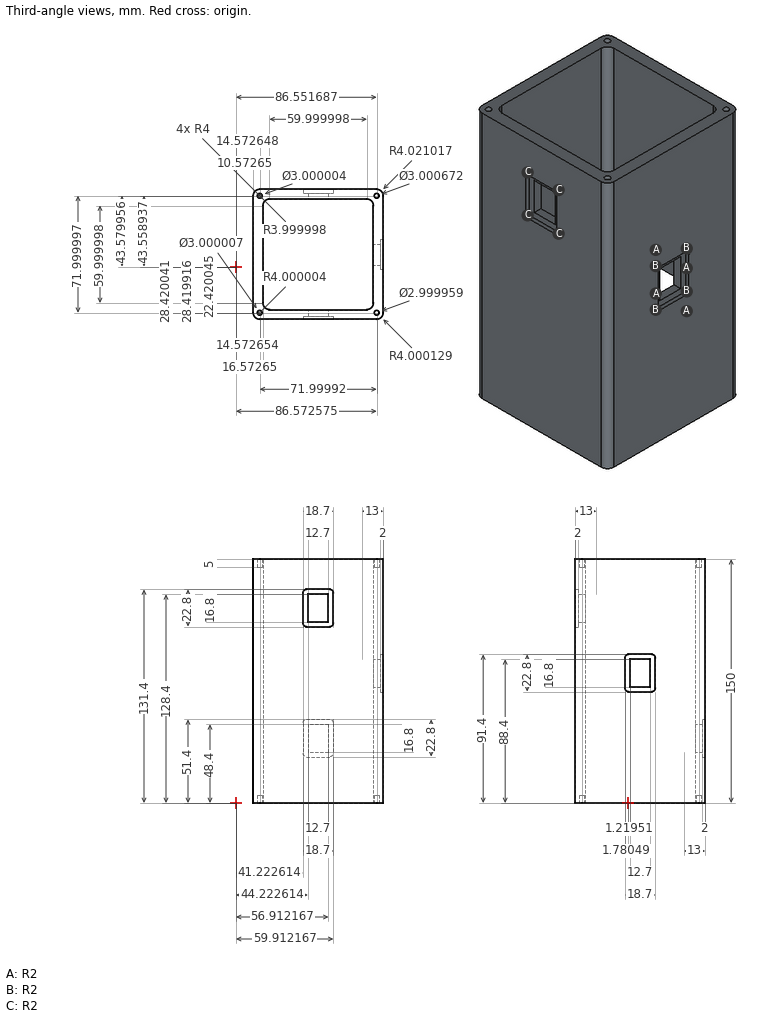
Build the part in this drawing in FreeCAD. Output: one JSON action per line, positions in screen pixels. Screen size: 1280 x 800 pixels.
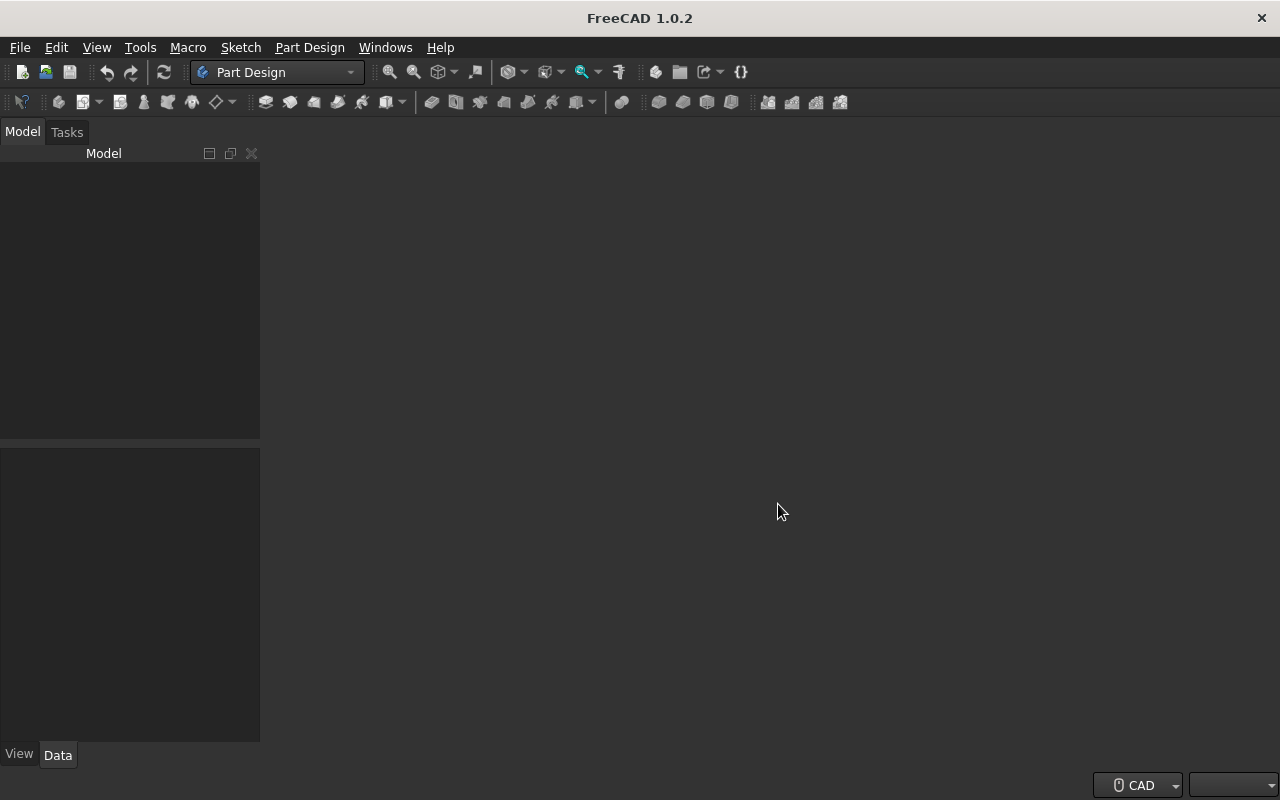
{"action": "left_click", "coordinate": [22, 72]}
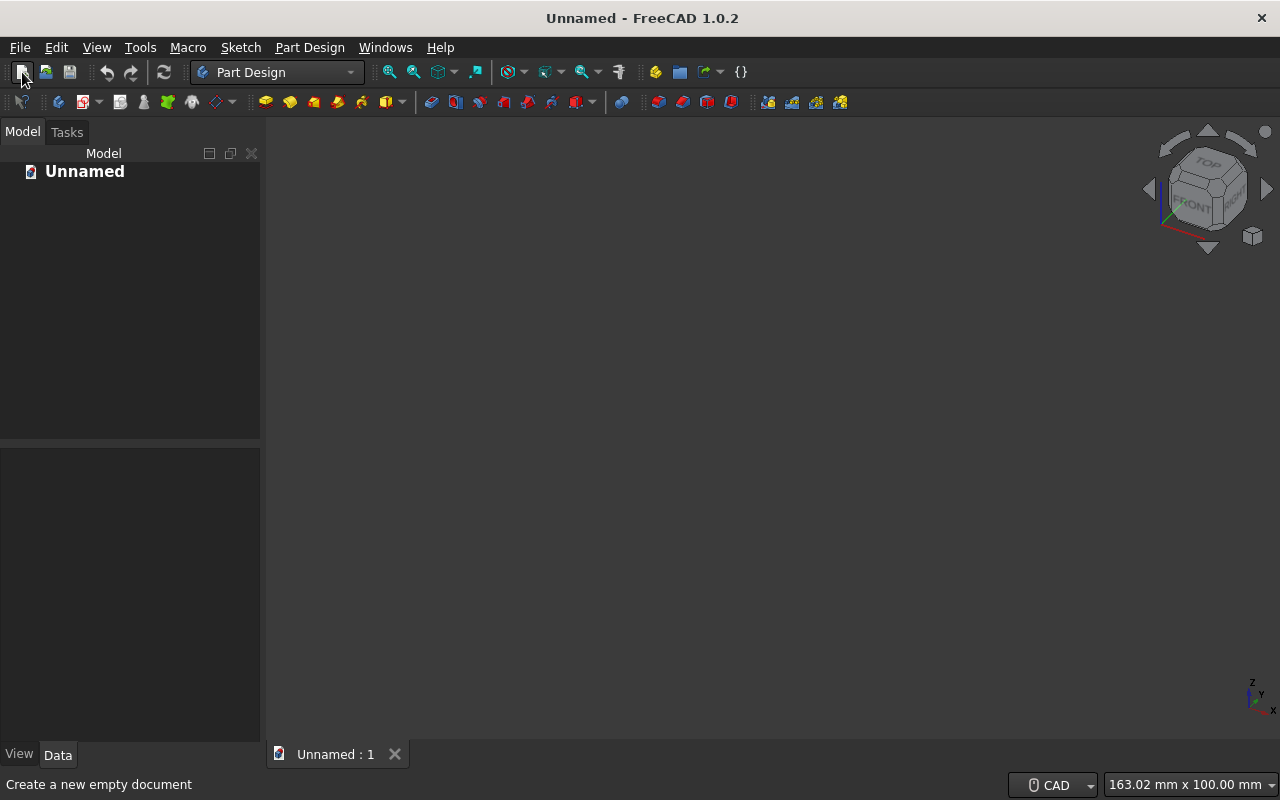
{"action": "left_click", "coordinate": [84, 102]}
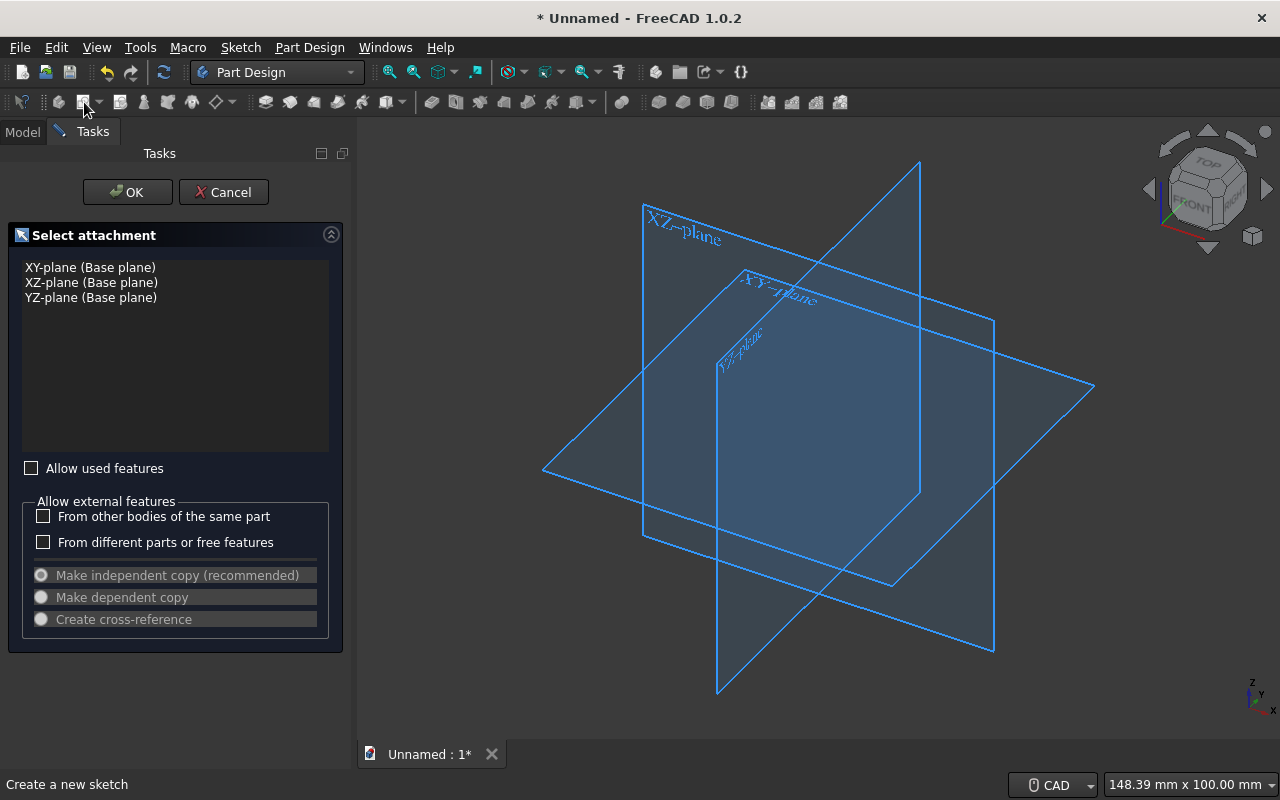
{"action": "left_click", "coordinate": [82, 268]}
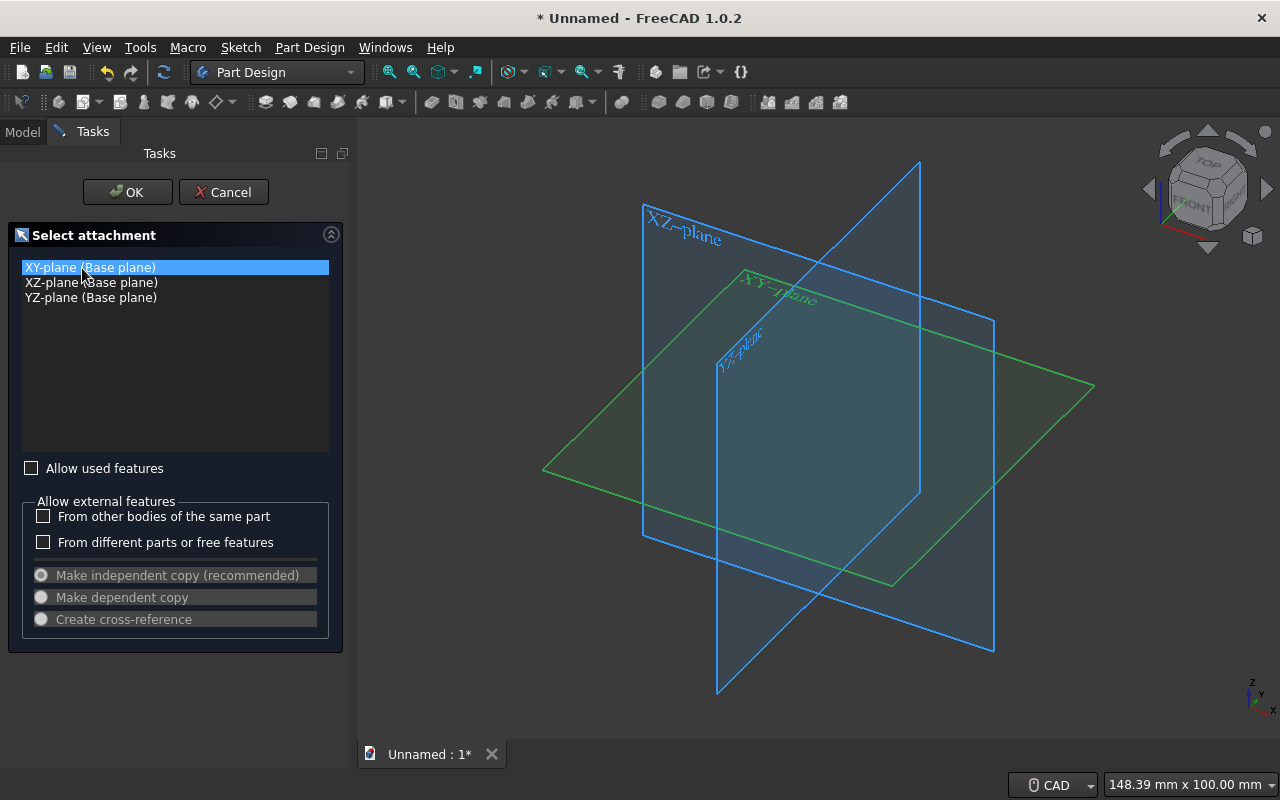
{"action": "left_click", "coordinate": [128, 192]}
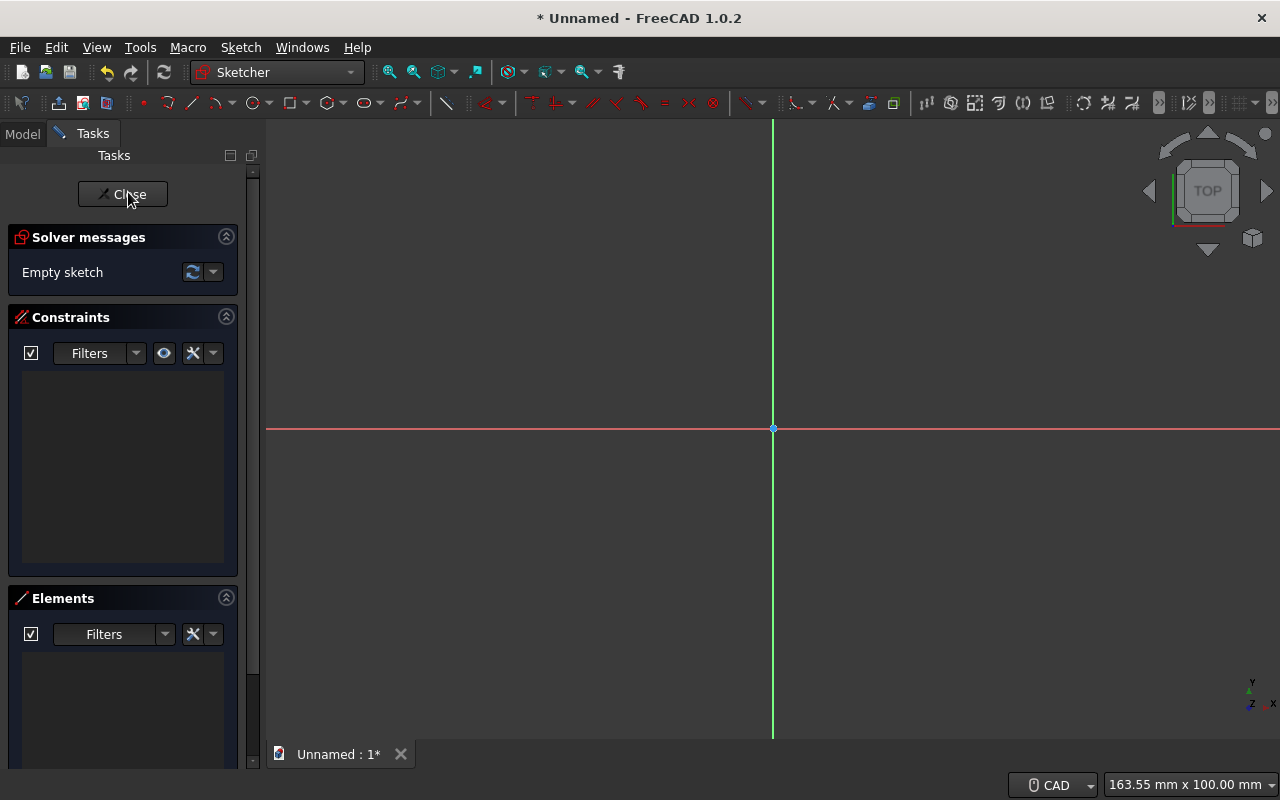
{"action": "scroll", "coordinate": [294, 525], "scroll_direction": "down", "scroll_amount": 2}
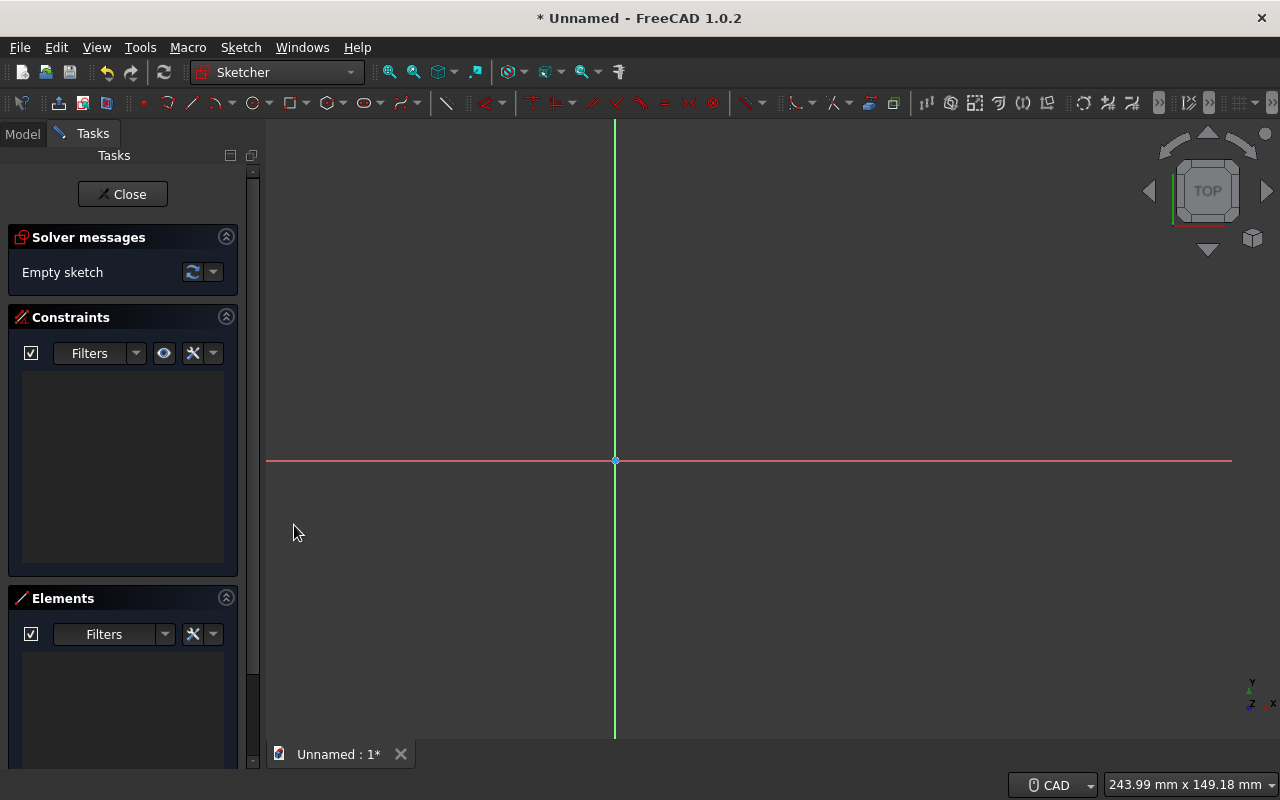
{"action": "left_click", "coordinate": [192, 104]}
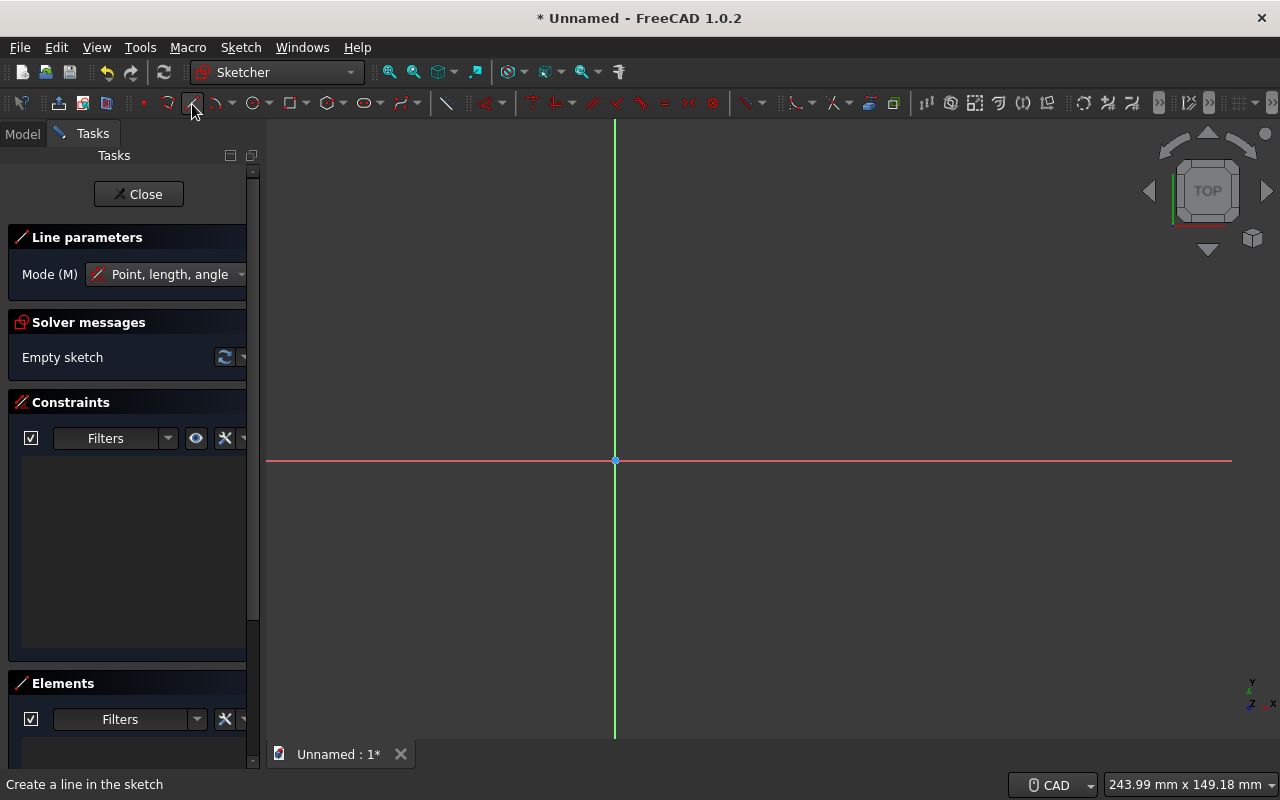
{"action": "left_click", "coordinate": [659, 280]}
{"action": "left_click", "coordinate": [659, 579]}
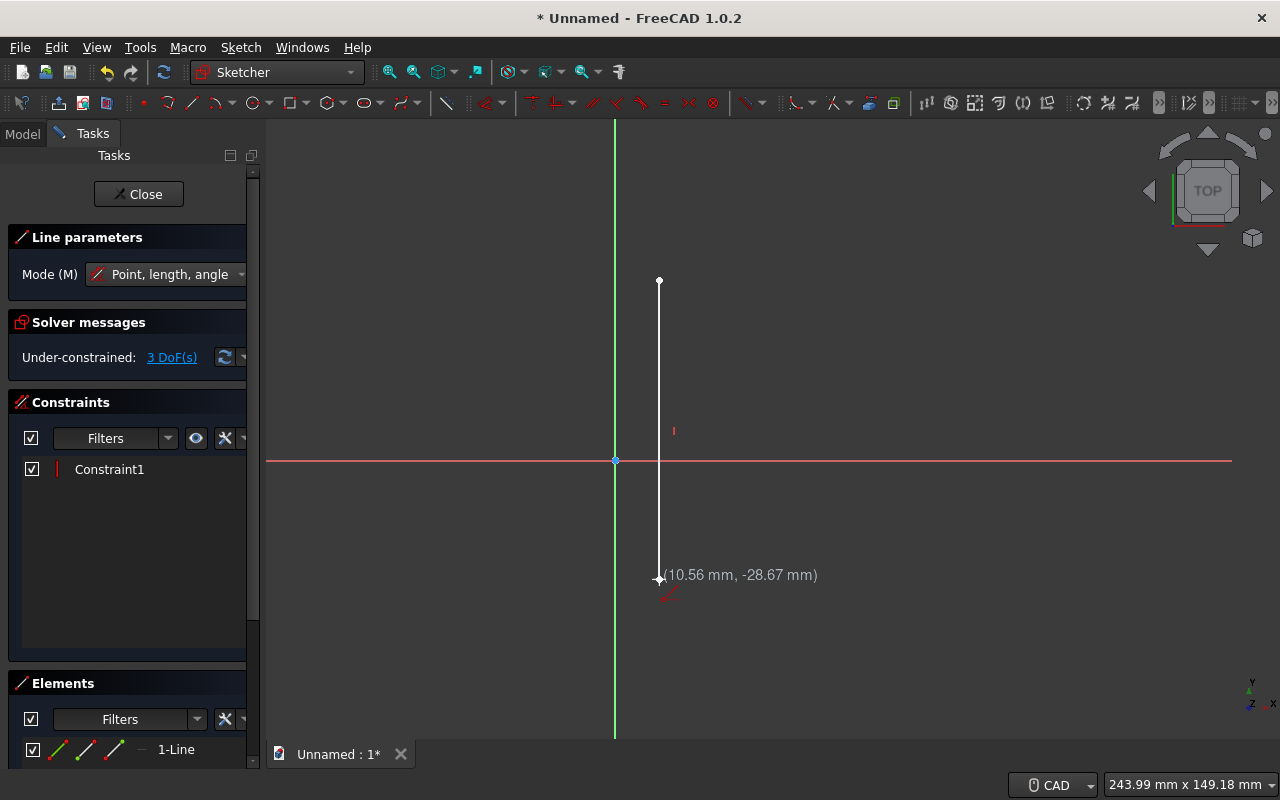
{"action": "left_click", "coordinate": [676, 596]}
{"action": "left_click", "coordinate": [975, 596]}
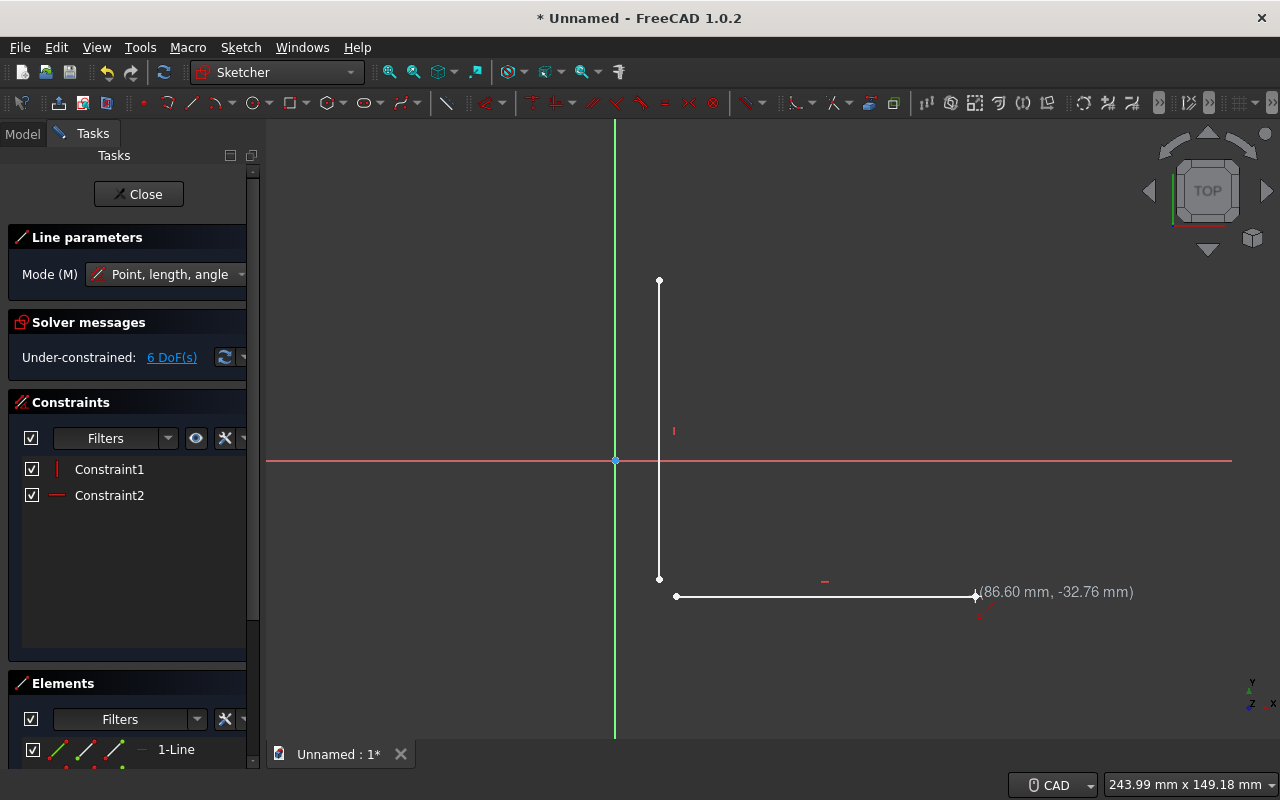
{"action": "left_click", "coordinate": [992, 579]}
{"action": "left_click", "coordinate": [992, 280]}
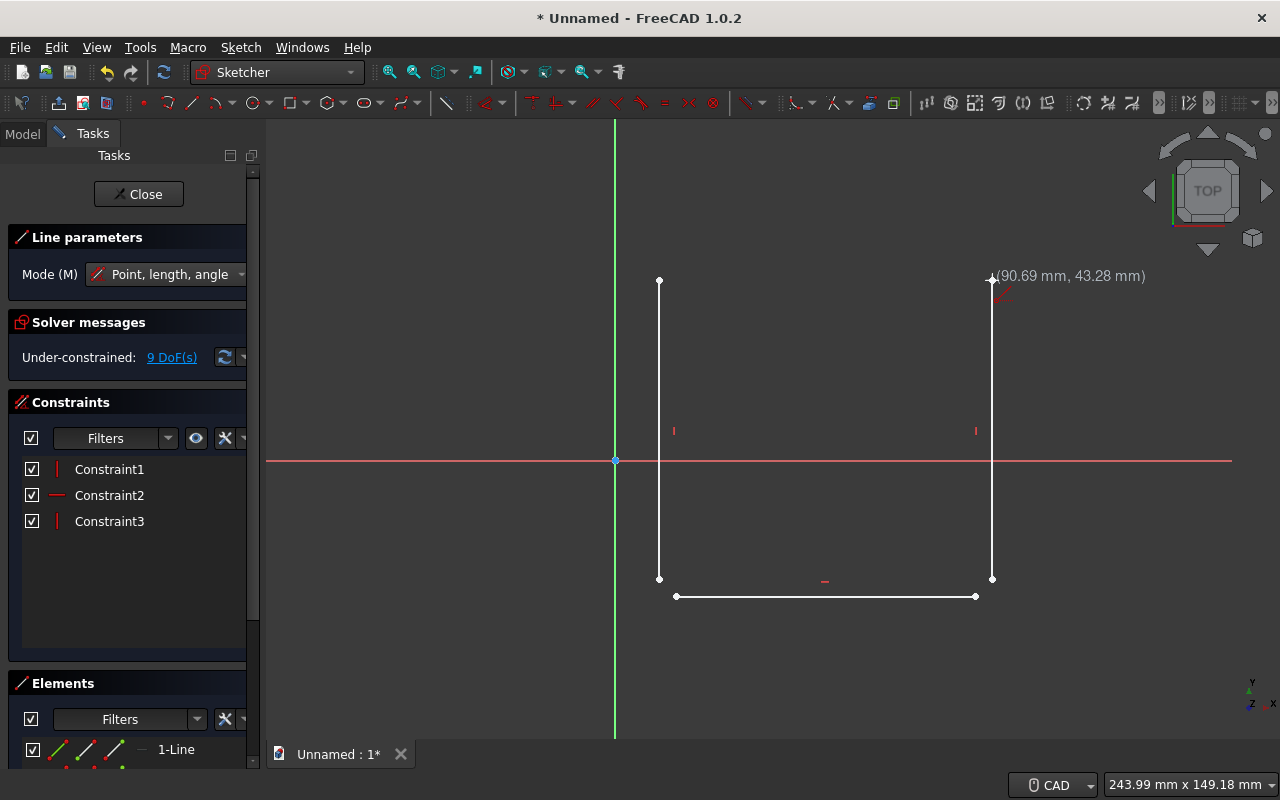
{"action": "left_click", "coordinate": [975, 263]}
{"action": "left_click", "coordinate": [676, 263]}